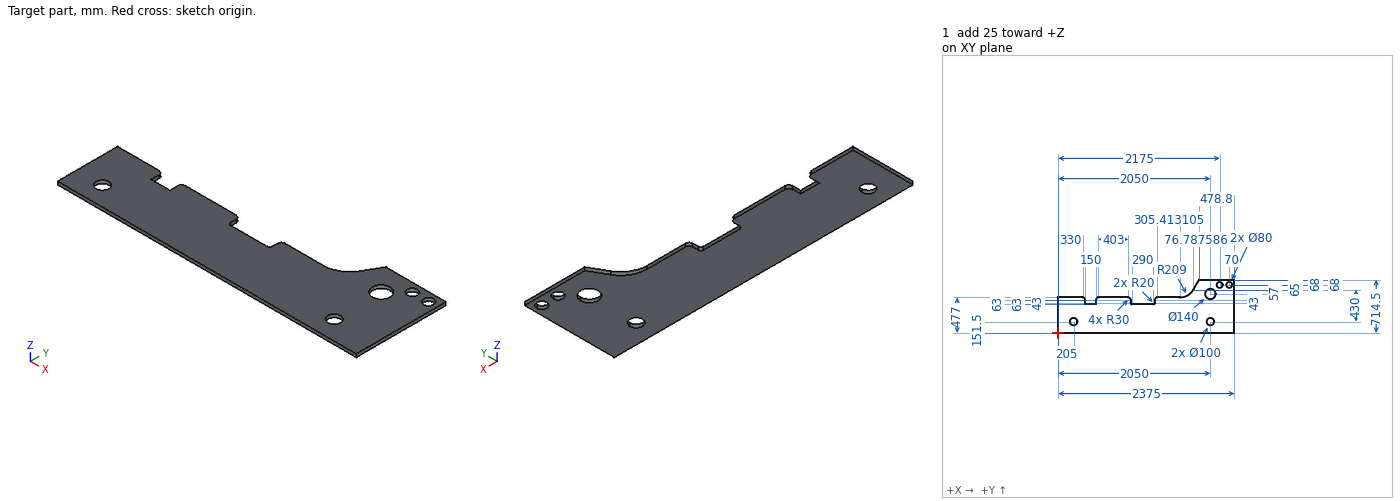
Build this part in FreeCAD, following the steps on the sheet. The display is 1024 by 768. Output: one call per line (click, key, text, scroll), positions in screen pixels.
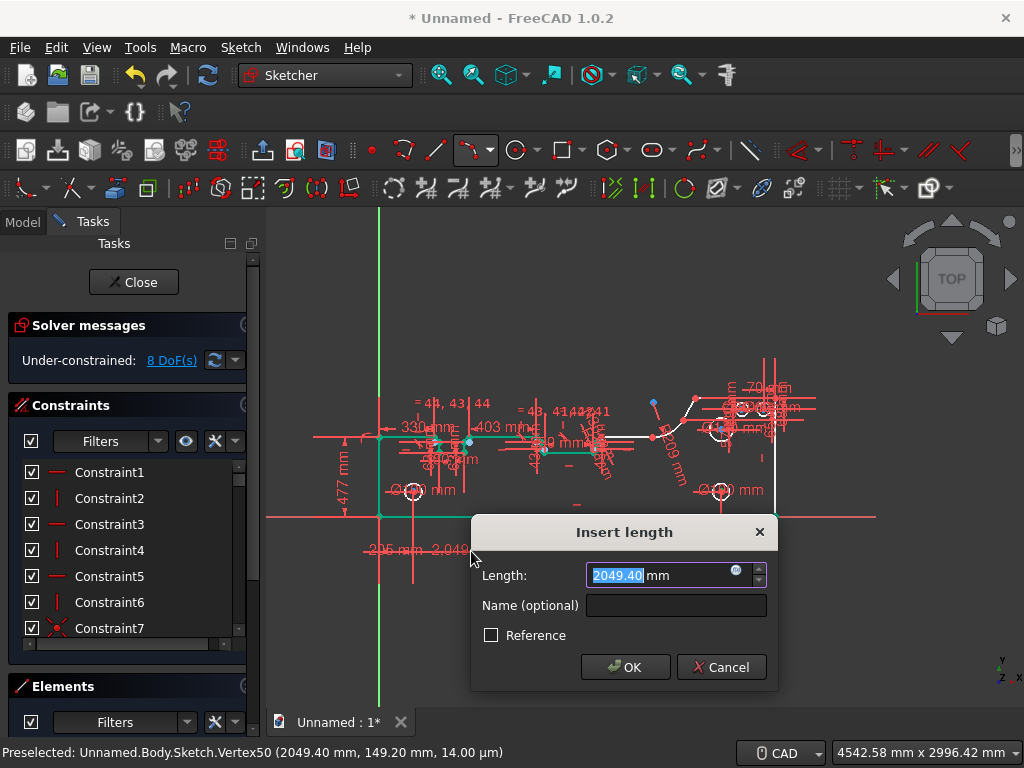
text(2050)
key(Return)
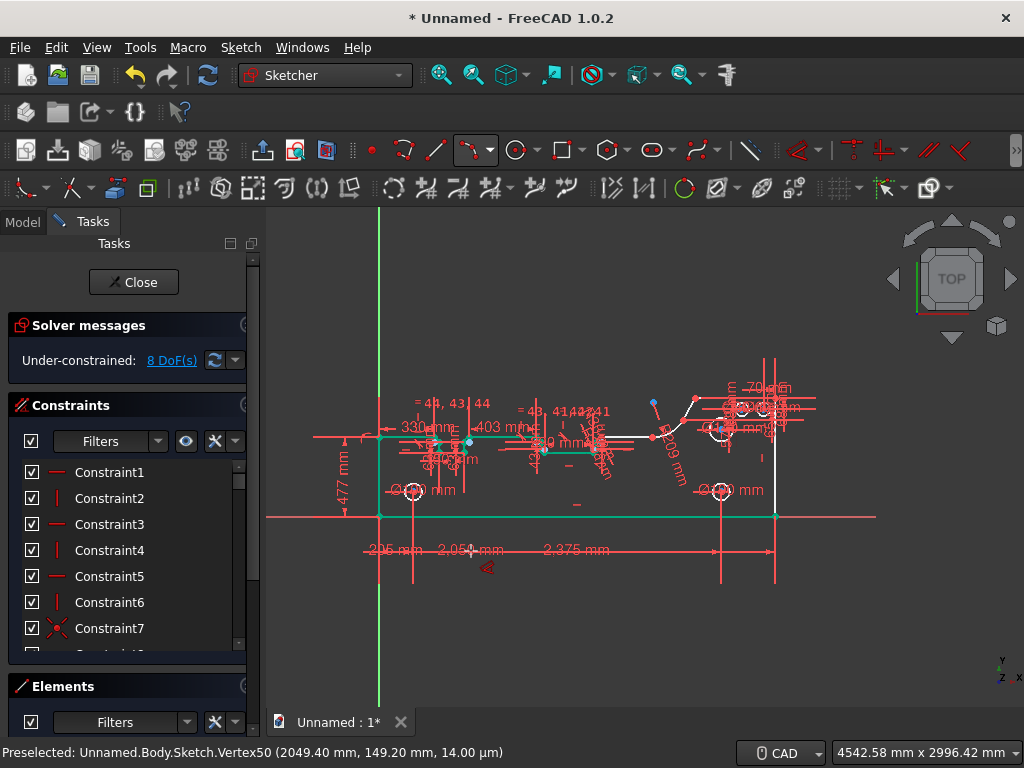
click(721, 430)
click(670, 551)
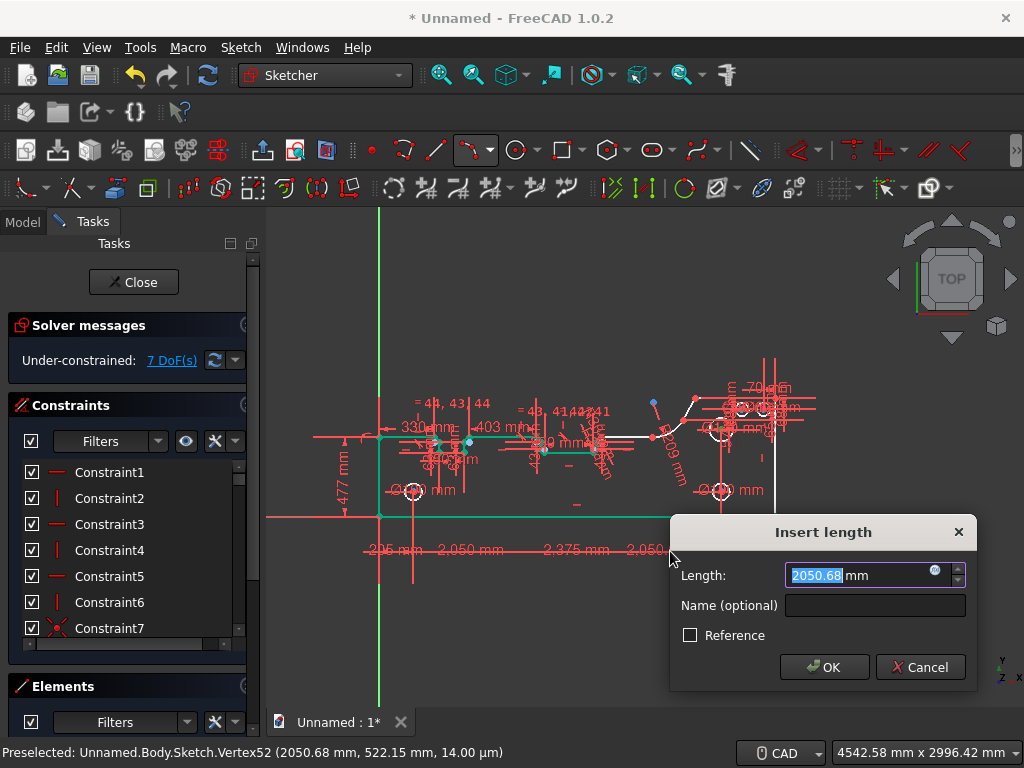
text(2050)
key(Return)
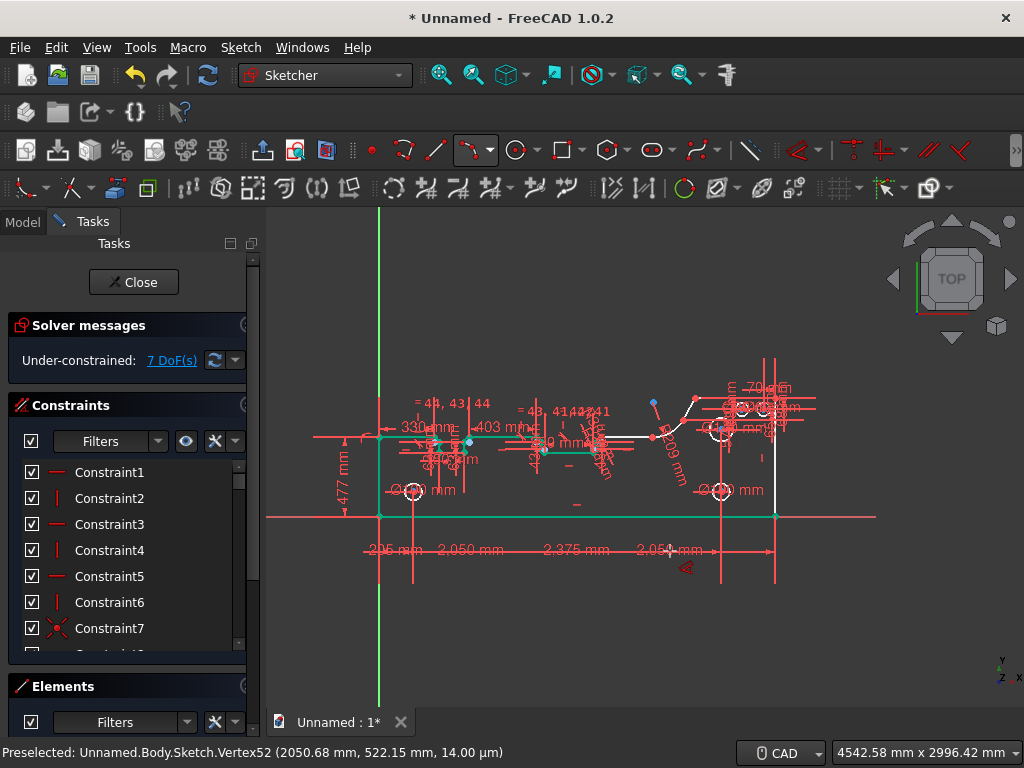
click(742, 409)
click(561, 375)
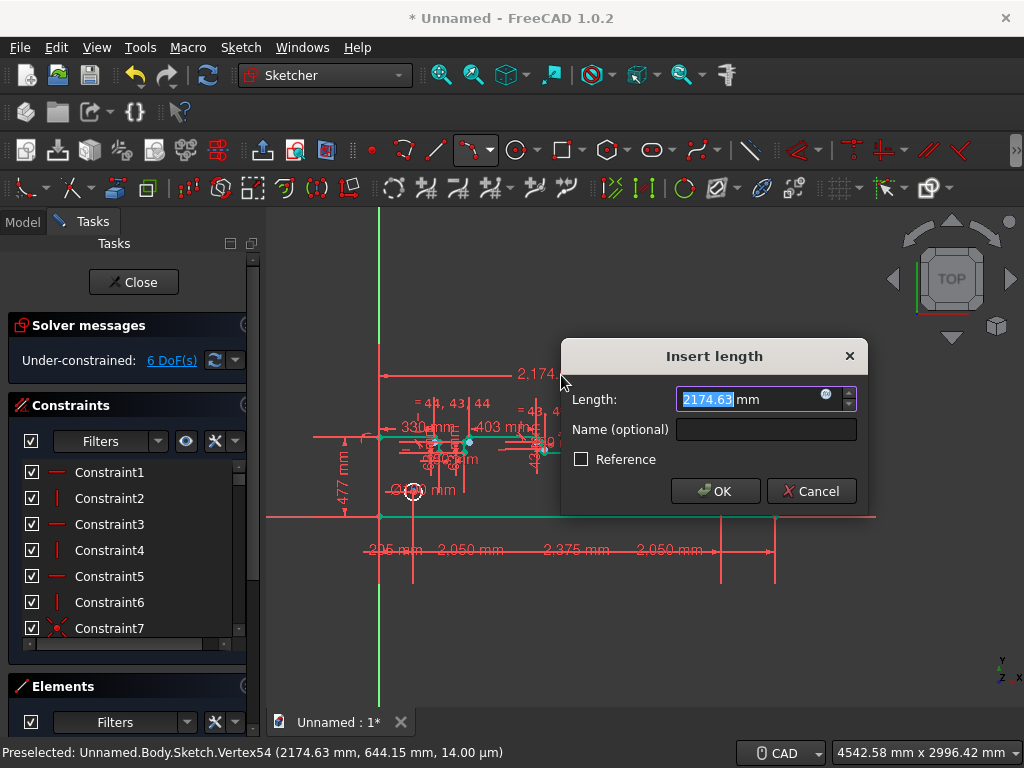
text(2175)
key(Return)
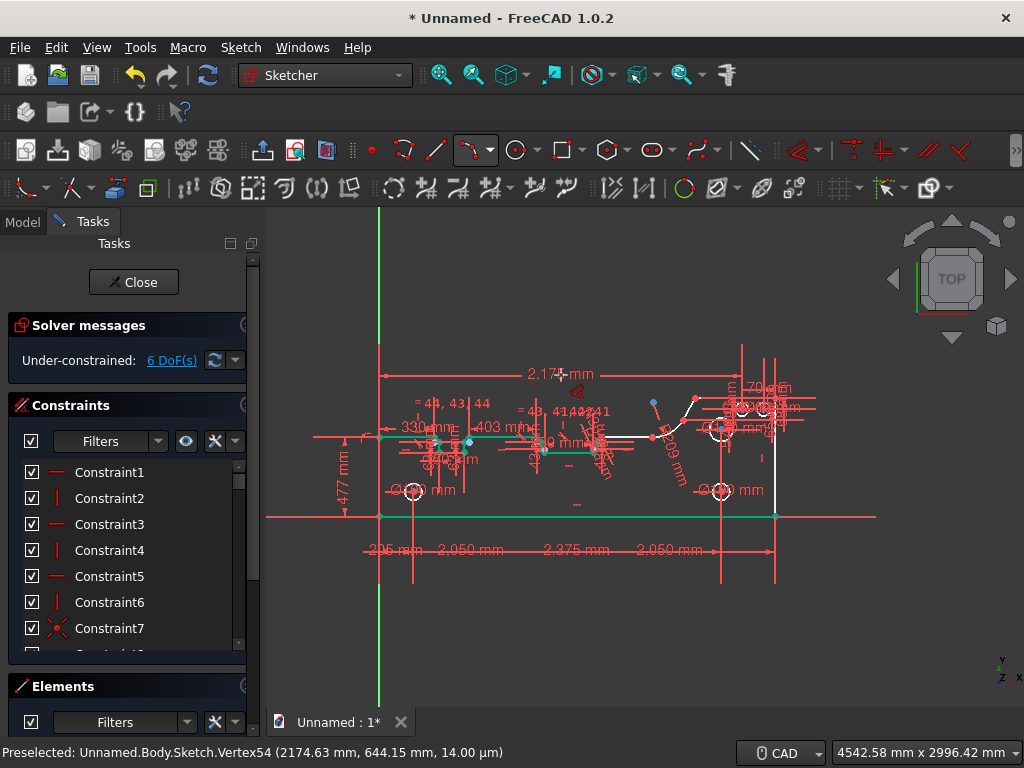
click(683, 420)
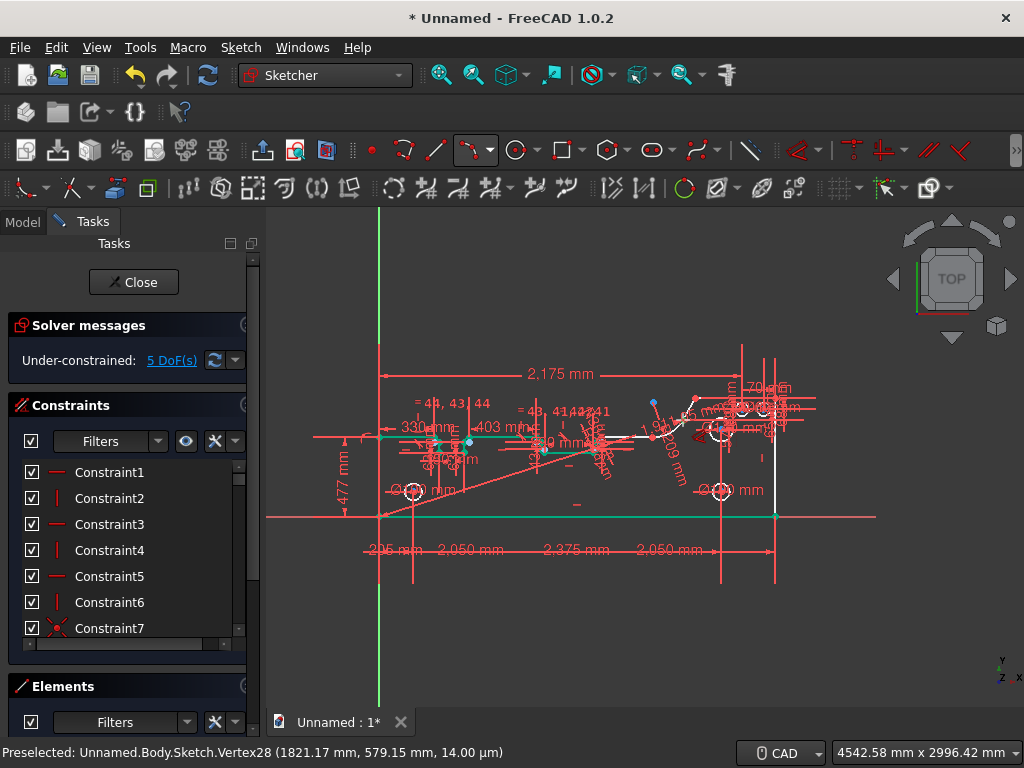
click(721, 492)
click(755, 456)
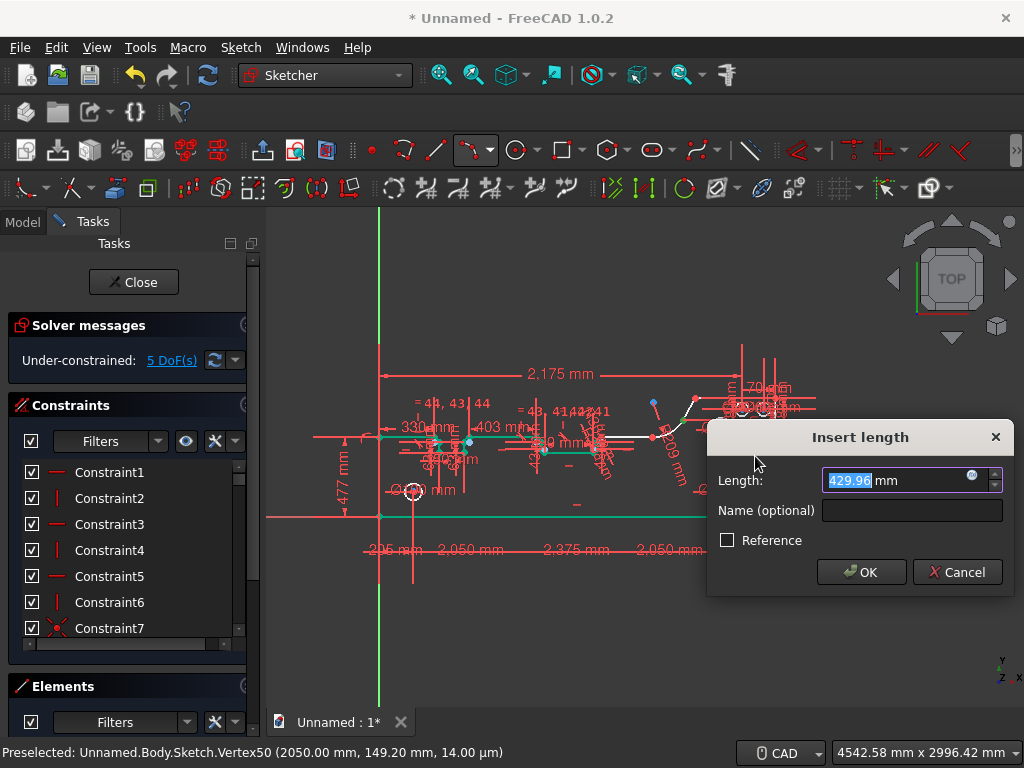
text(430)
key(Return)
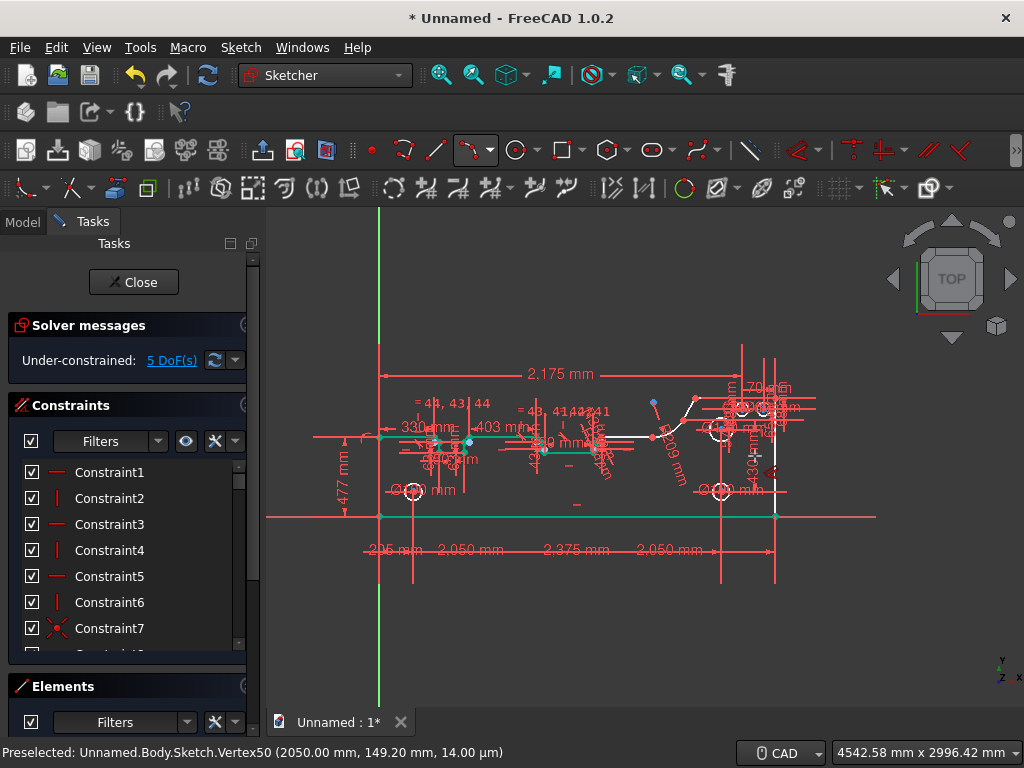
click(775, 481)
click(809, 485)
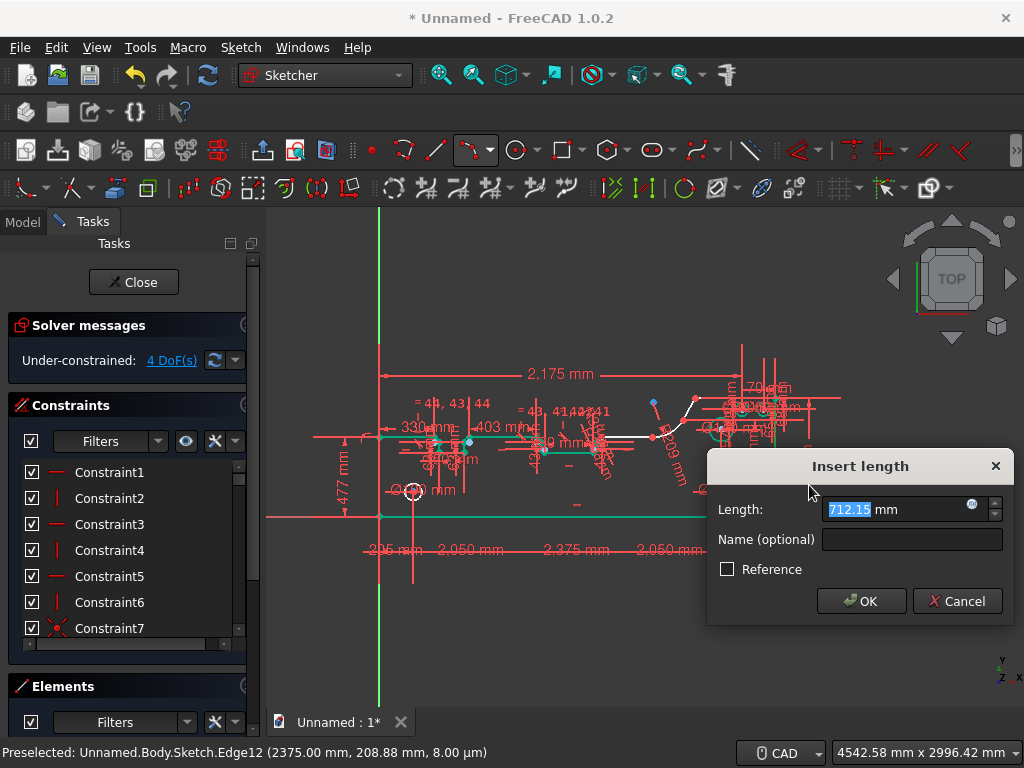
text(714.5)
key(Return)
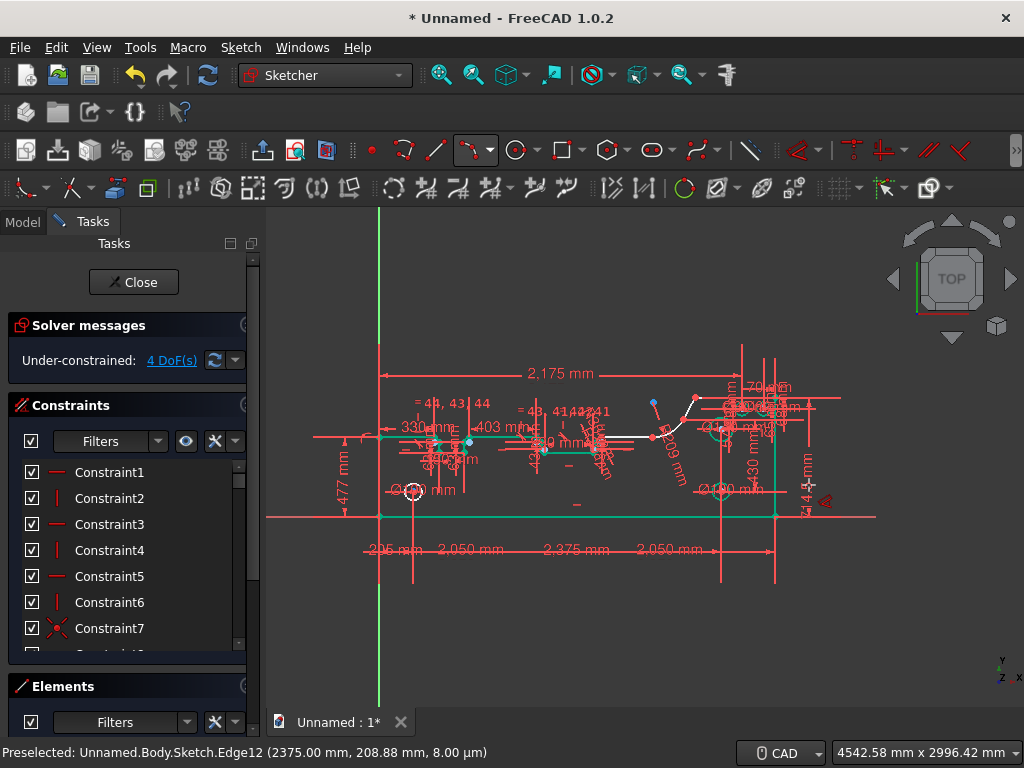
click(719, 398)
click(735, 364)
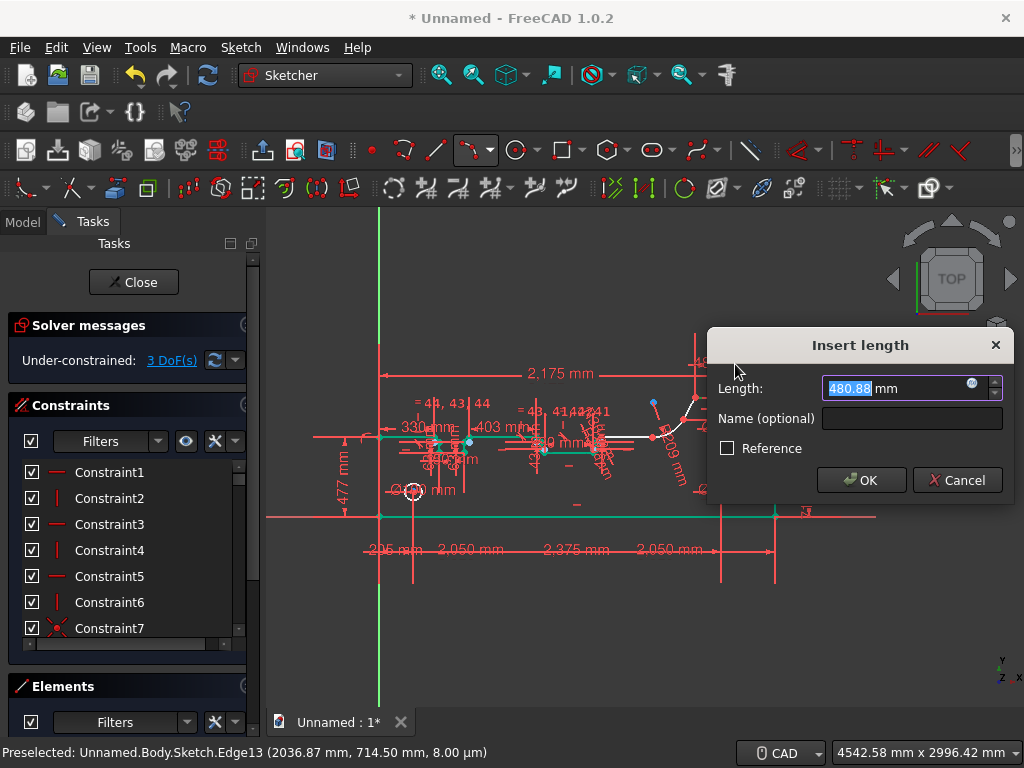
text(478.8)
key(Return)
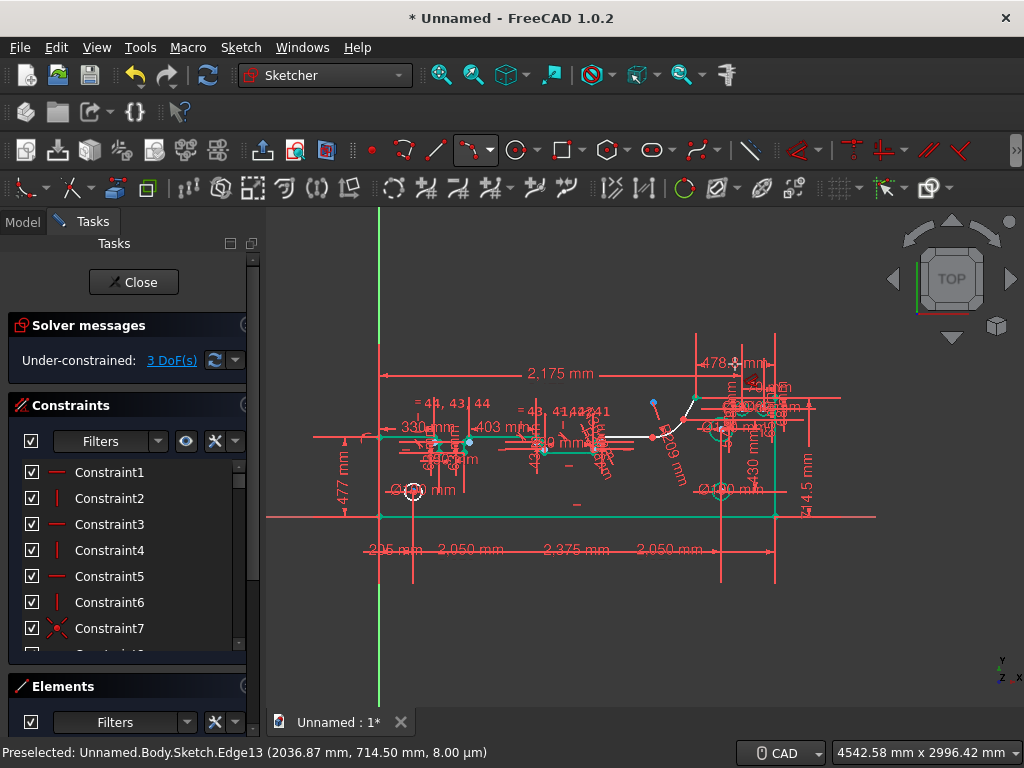
scroll(413, 492, up, 3)